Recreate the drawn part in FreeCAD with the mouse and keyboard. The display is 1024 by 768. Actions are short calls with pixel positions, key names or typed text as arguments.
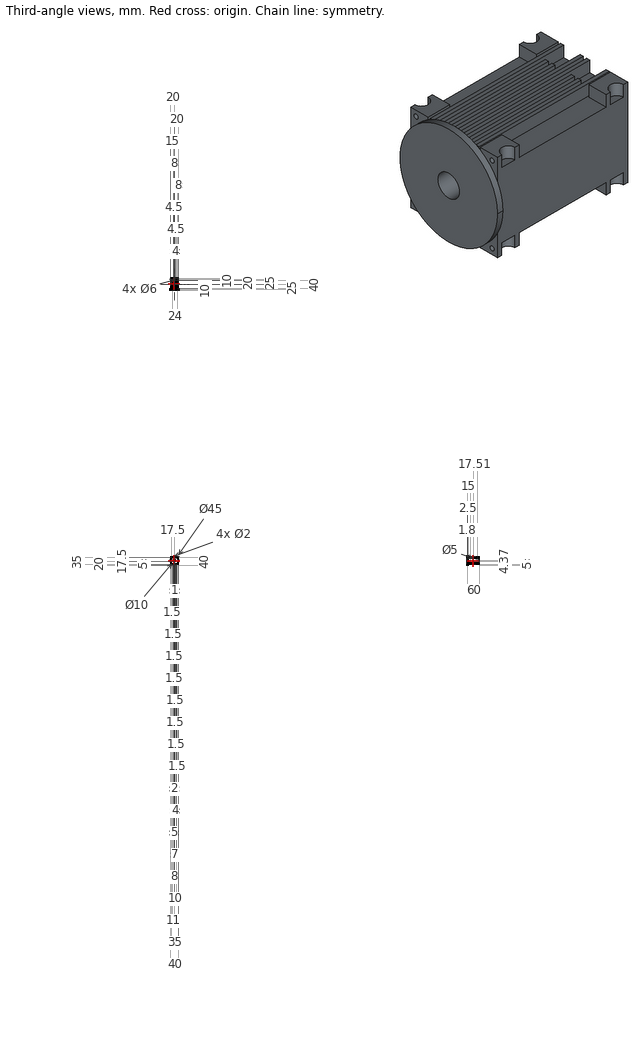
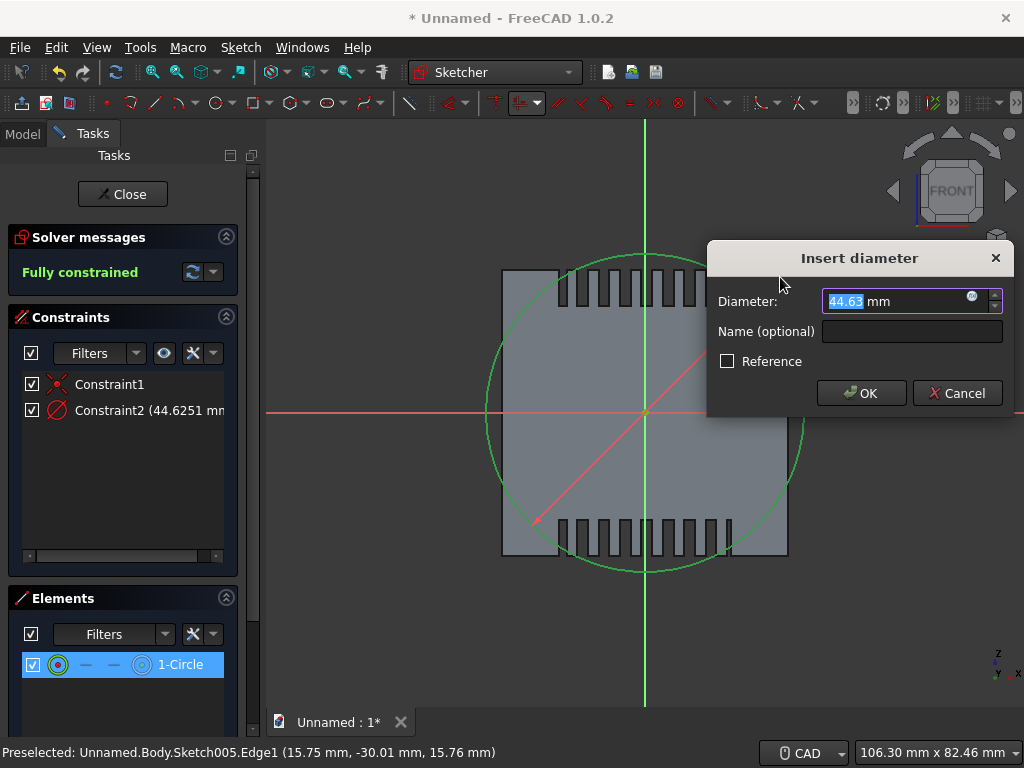
text(45)
key(Return)
key(Escape)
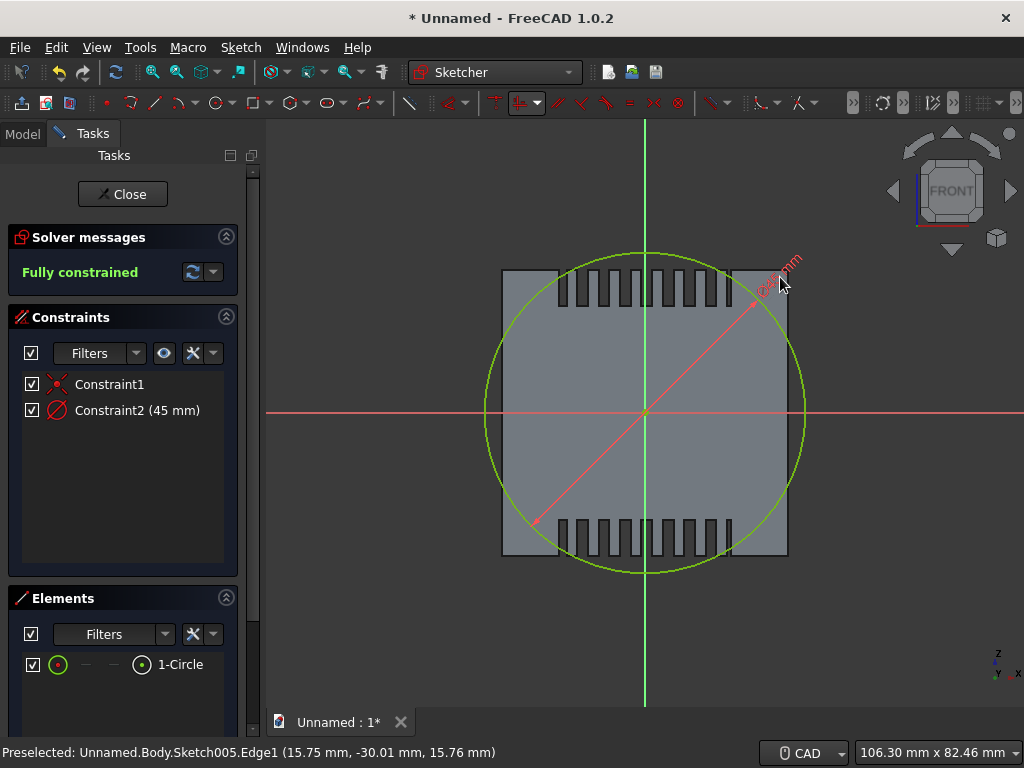
click(123, 194)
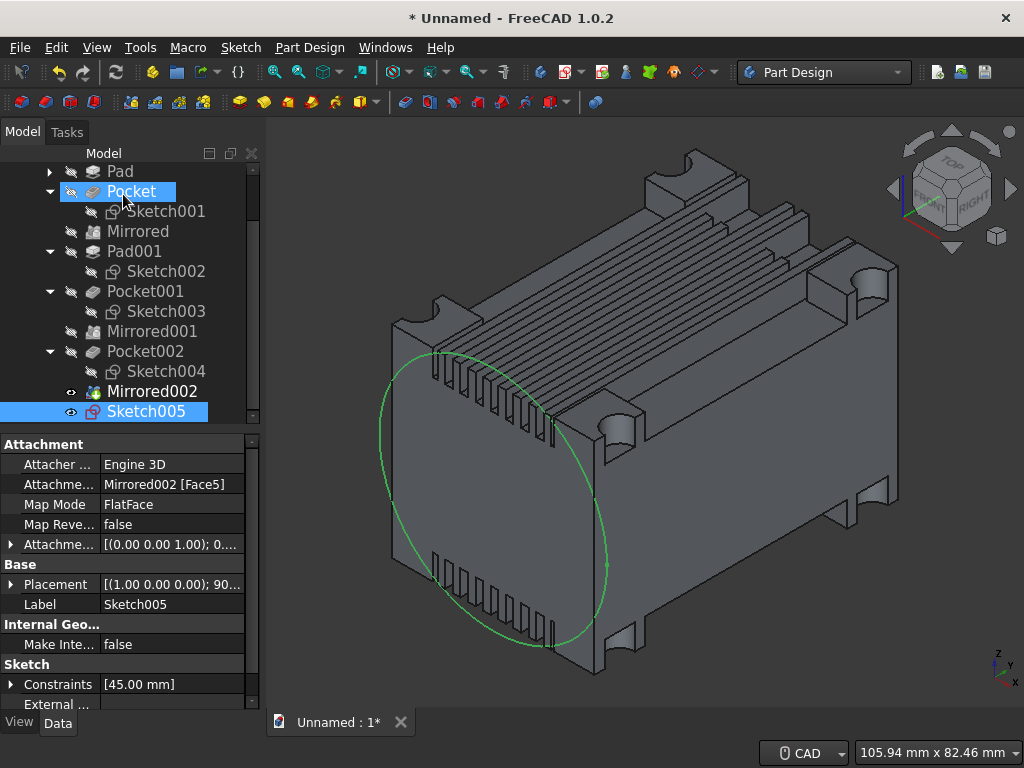
click(240, 102)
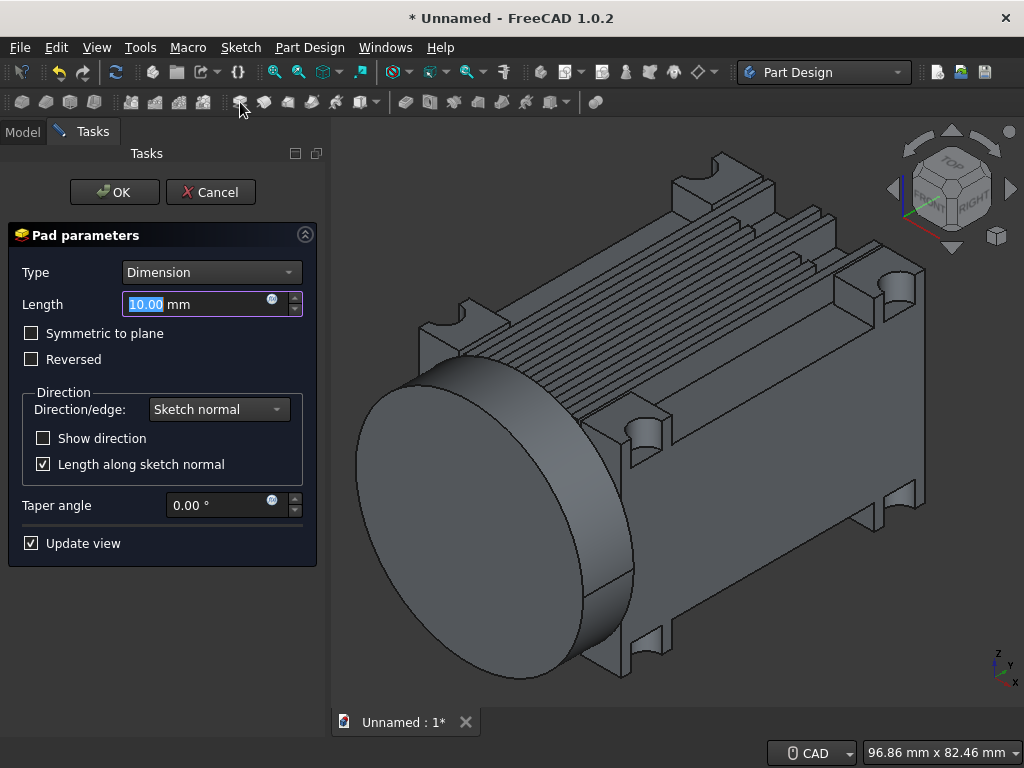
text(2.5)
key(Tab)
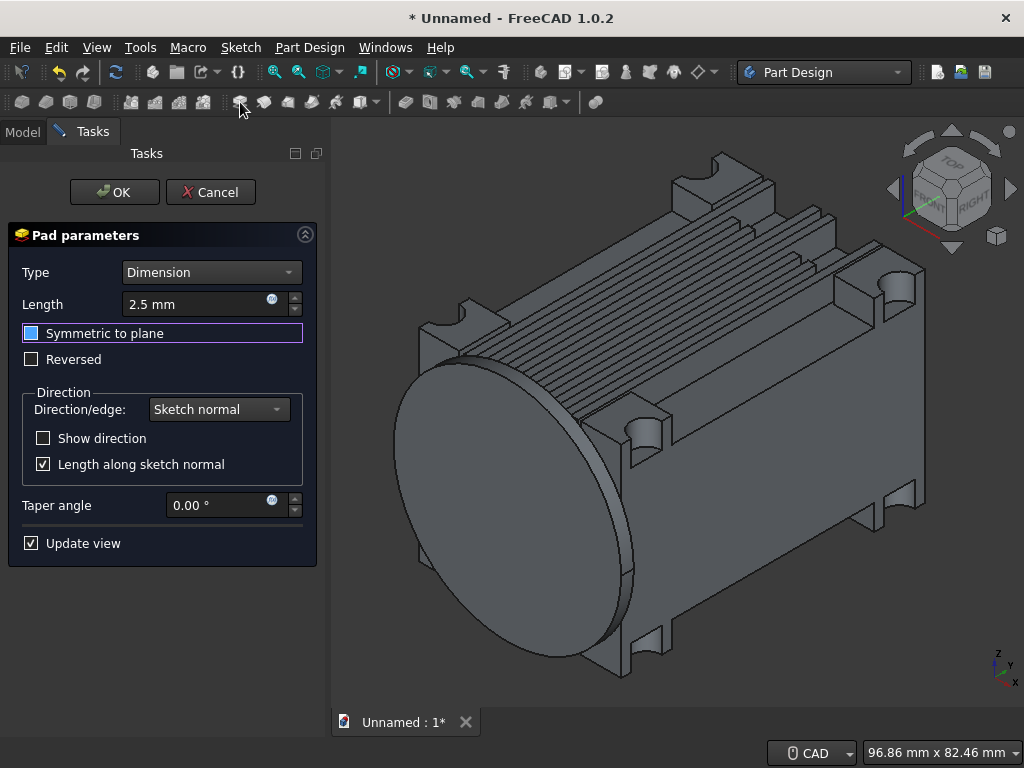
click(115, 192)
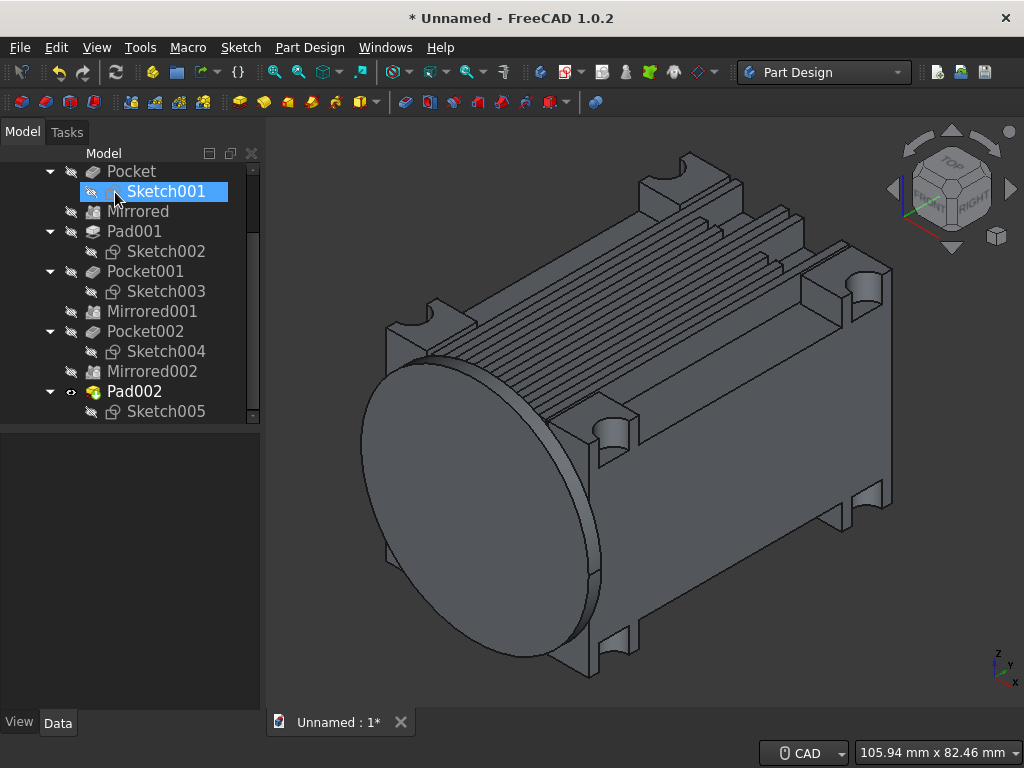
click(475, 509)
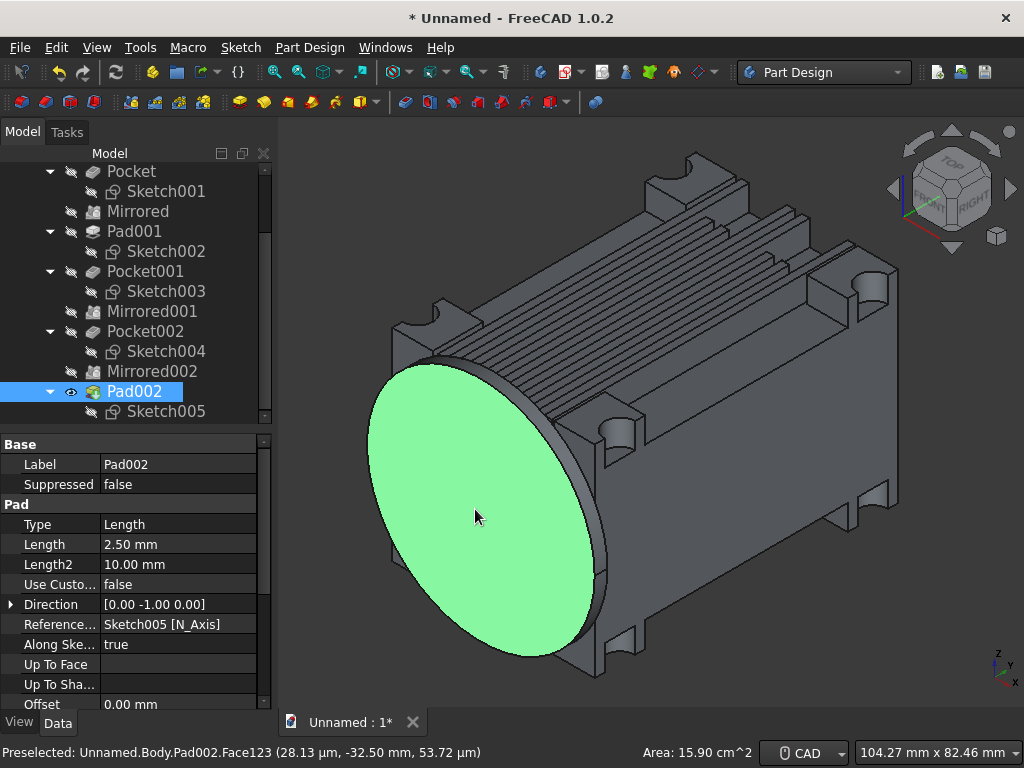
click(566, 72)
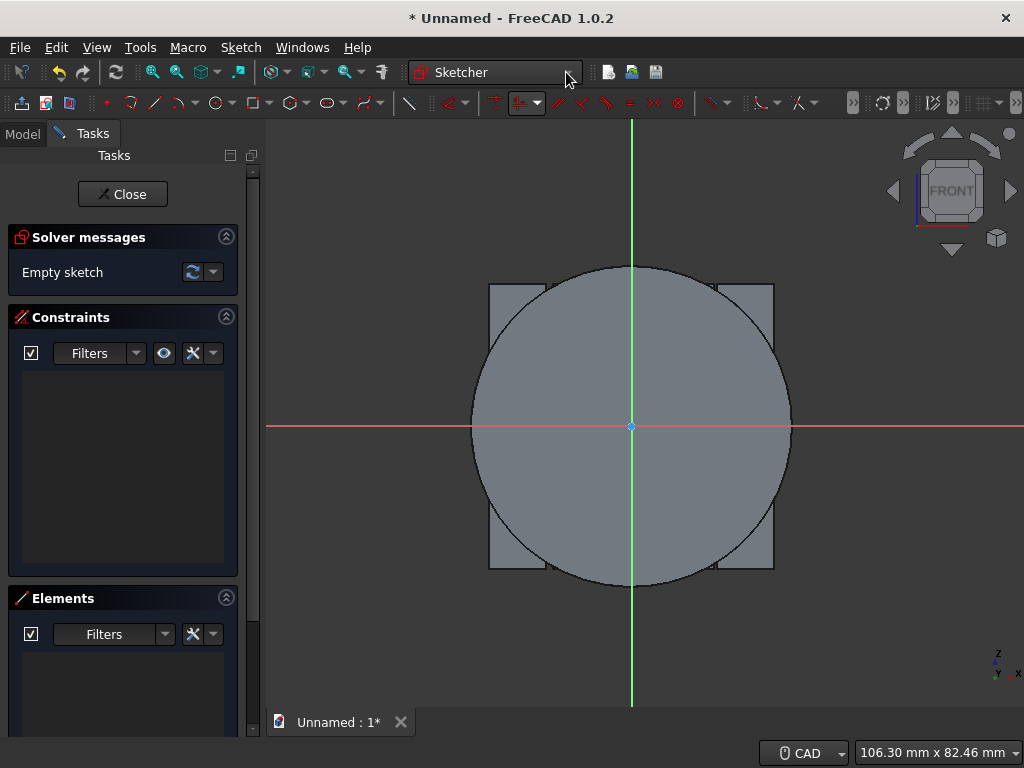
scroll(645, 430, up, 8)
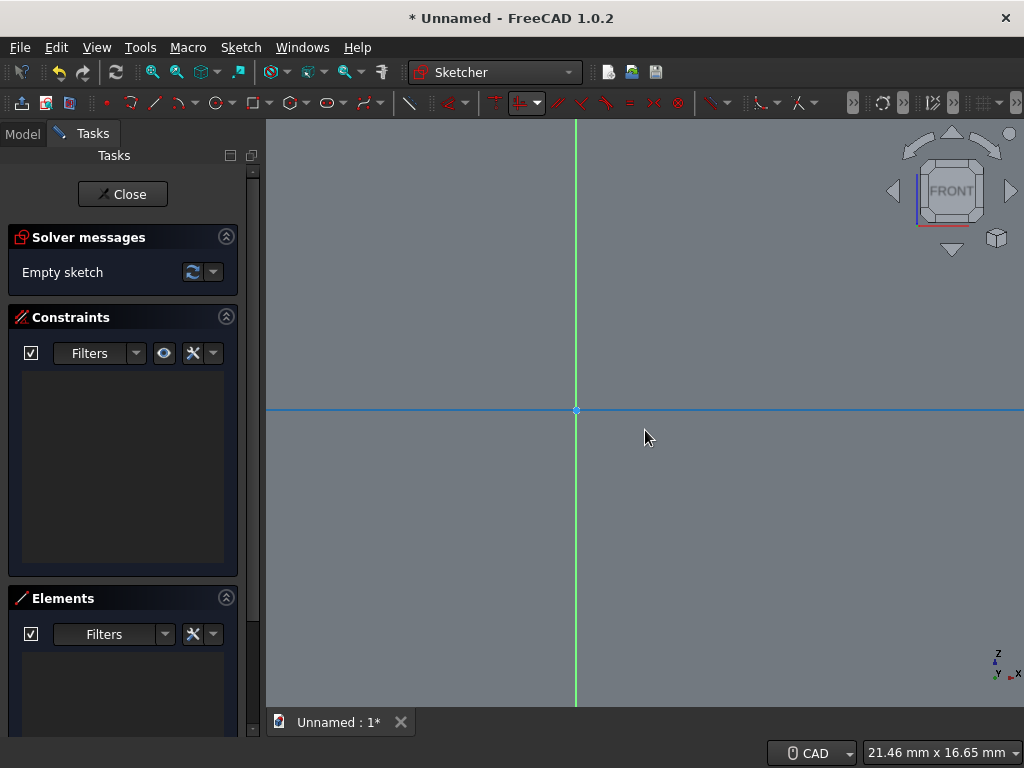
click(216, 104)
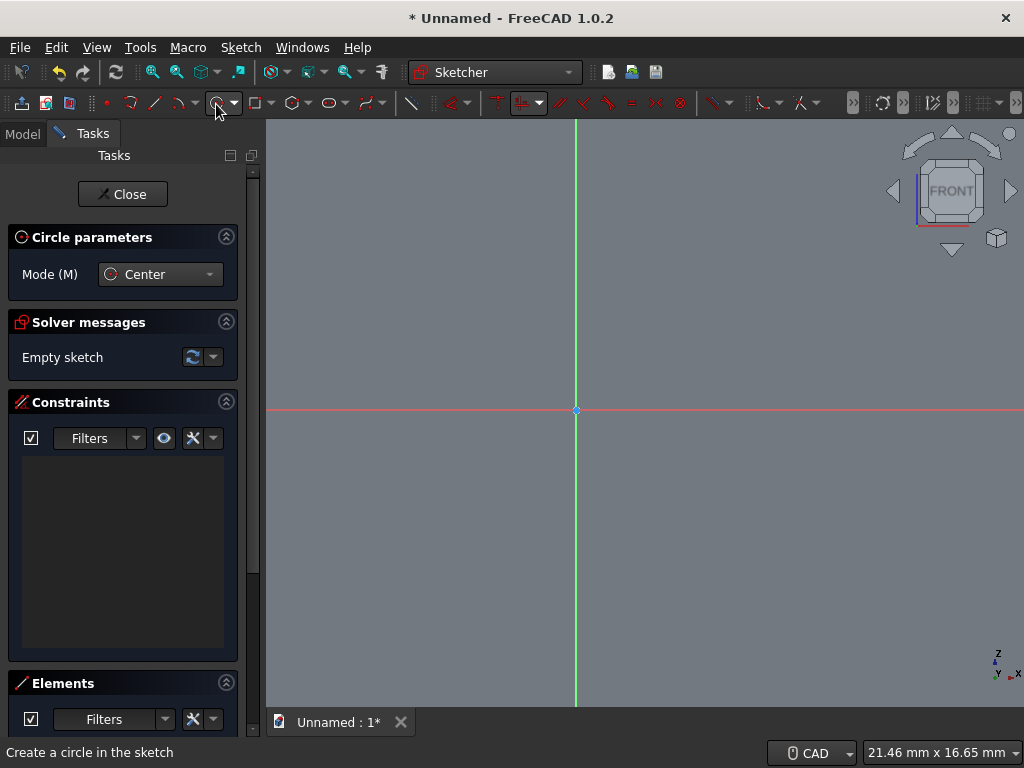
click(576, 410)
click(701, 286)
key(Escape)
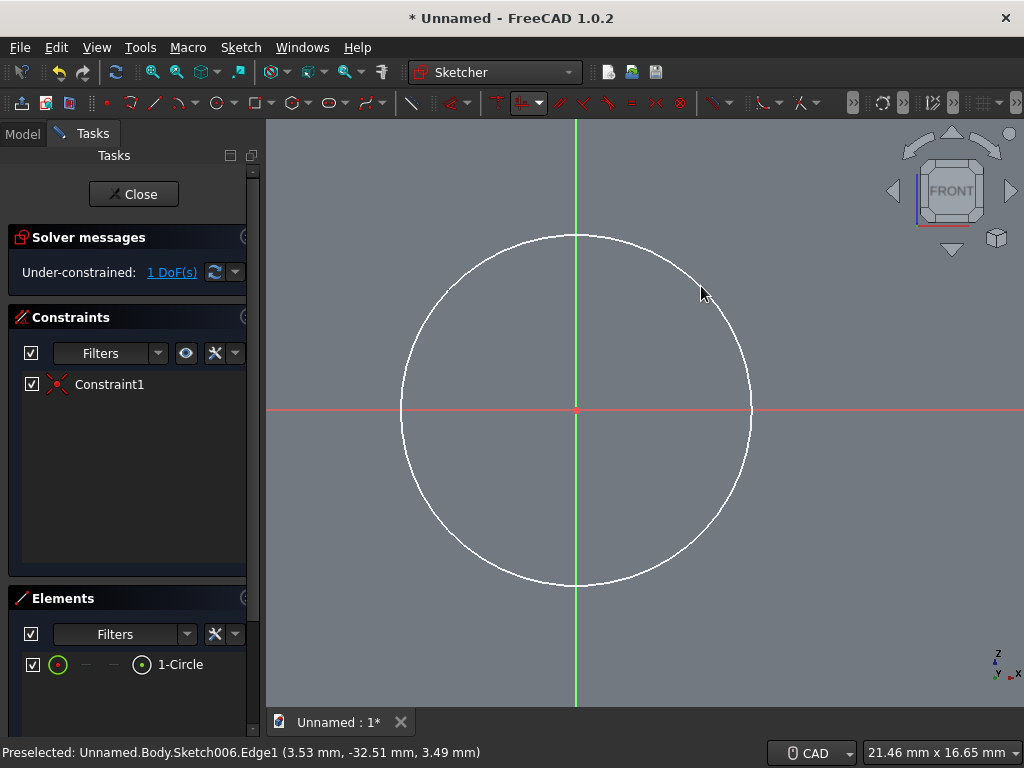
click(450, 104)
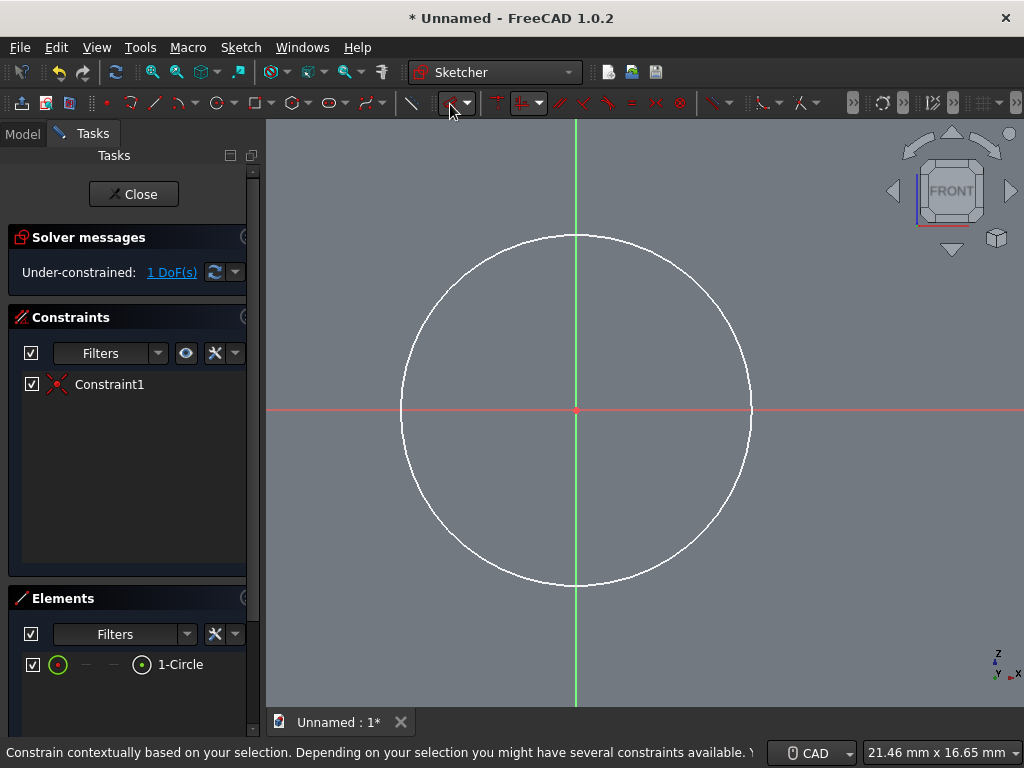
click(700, 286)
click(723, 263)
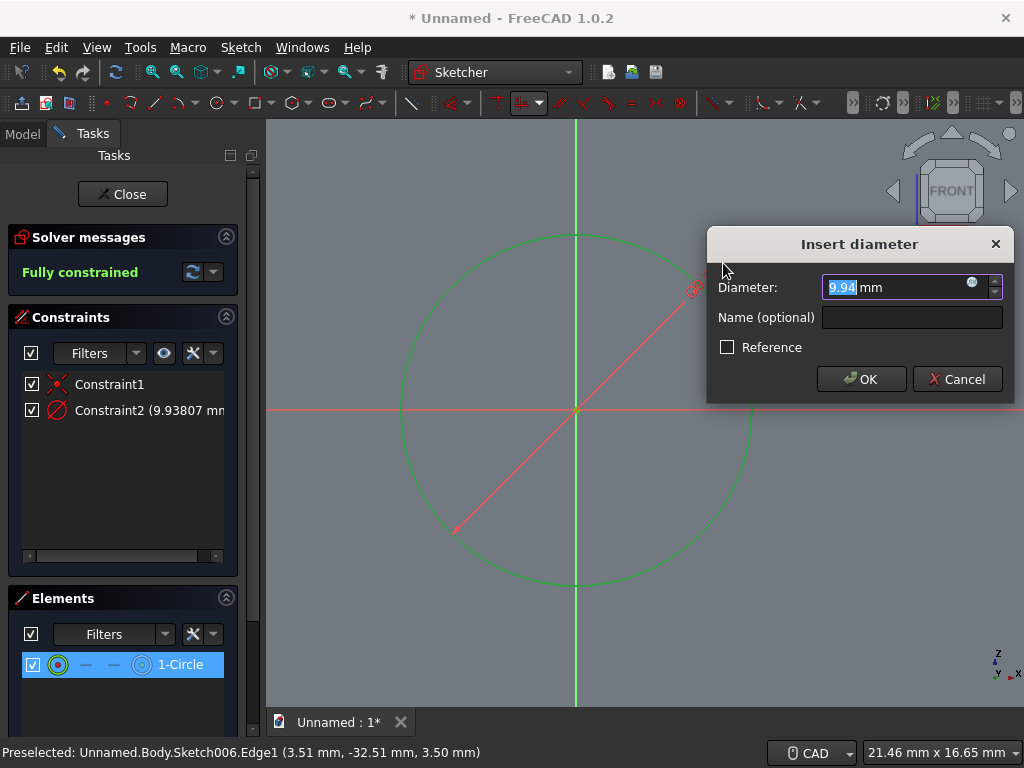
text(10)
key(Return)
key(Escape)